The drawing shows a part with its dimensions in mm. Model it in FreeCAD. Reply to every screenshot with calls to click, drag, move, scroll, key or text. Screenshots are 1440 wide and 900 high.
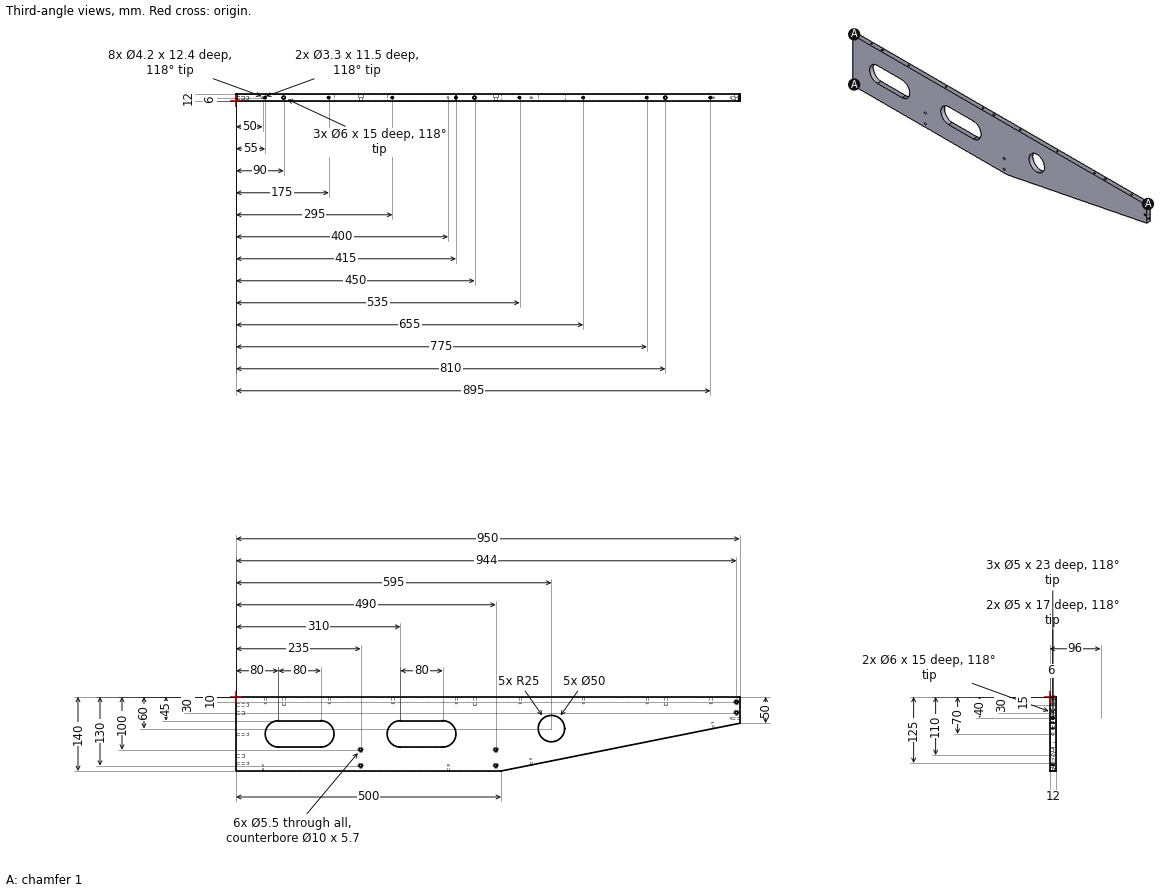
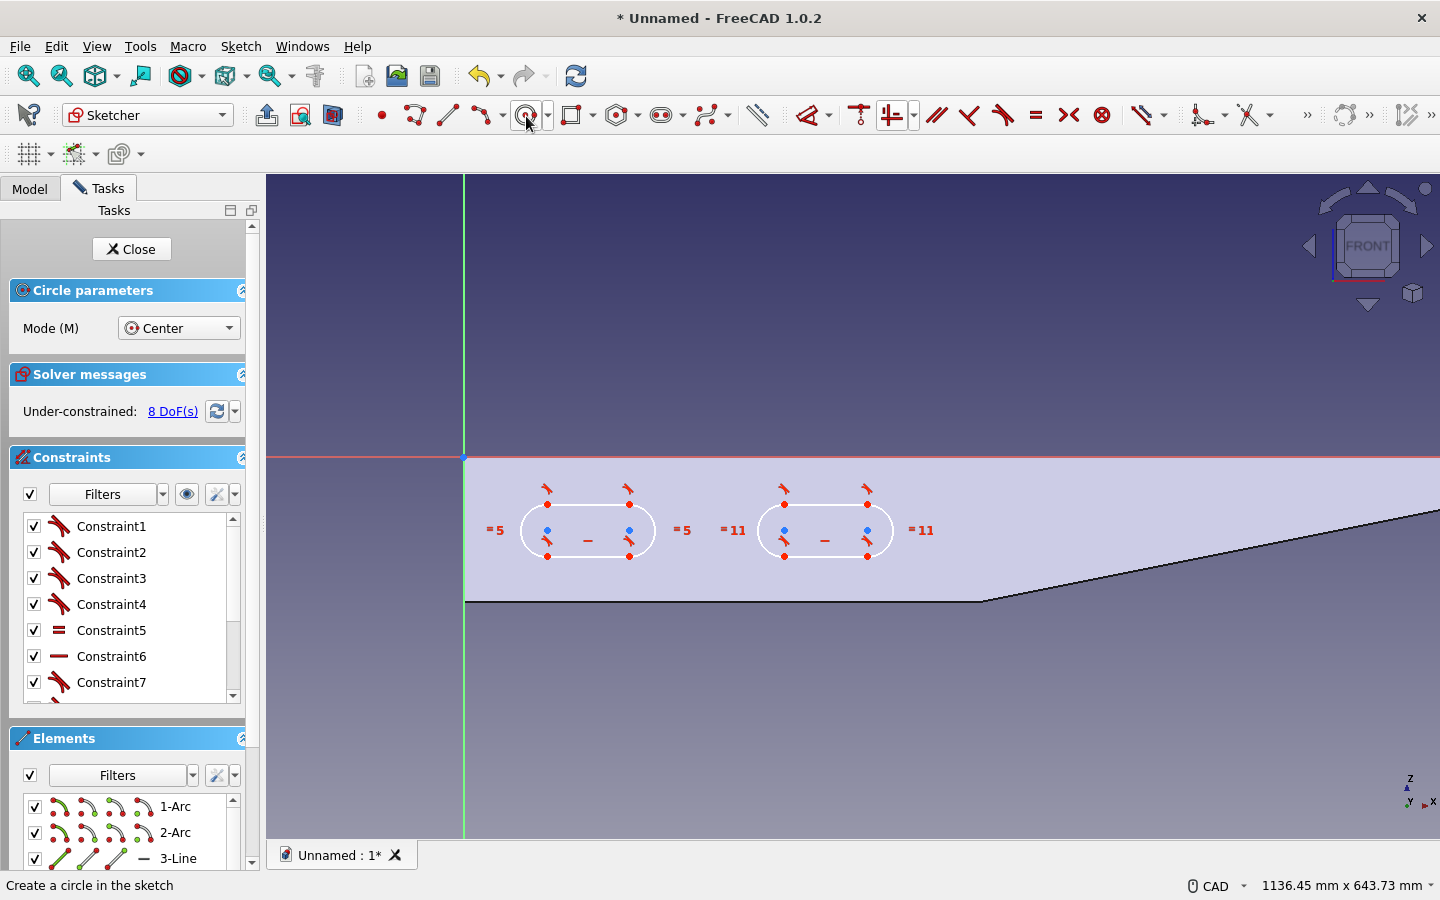
click(1079, 519)
move(1097, 501)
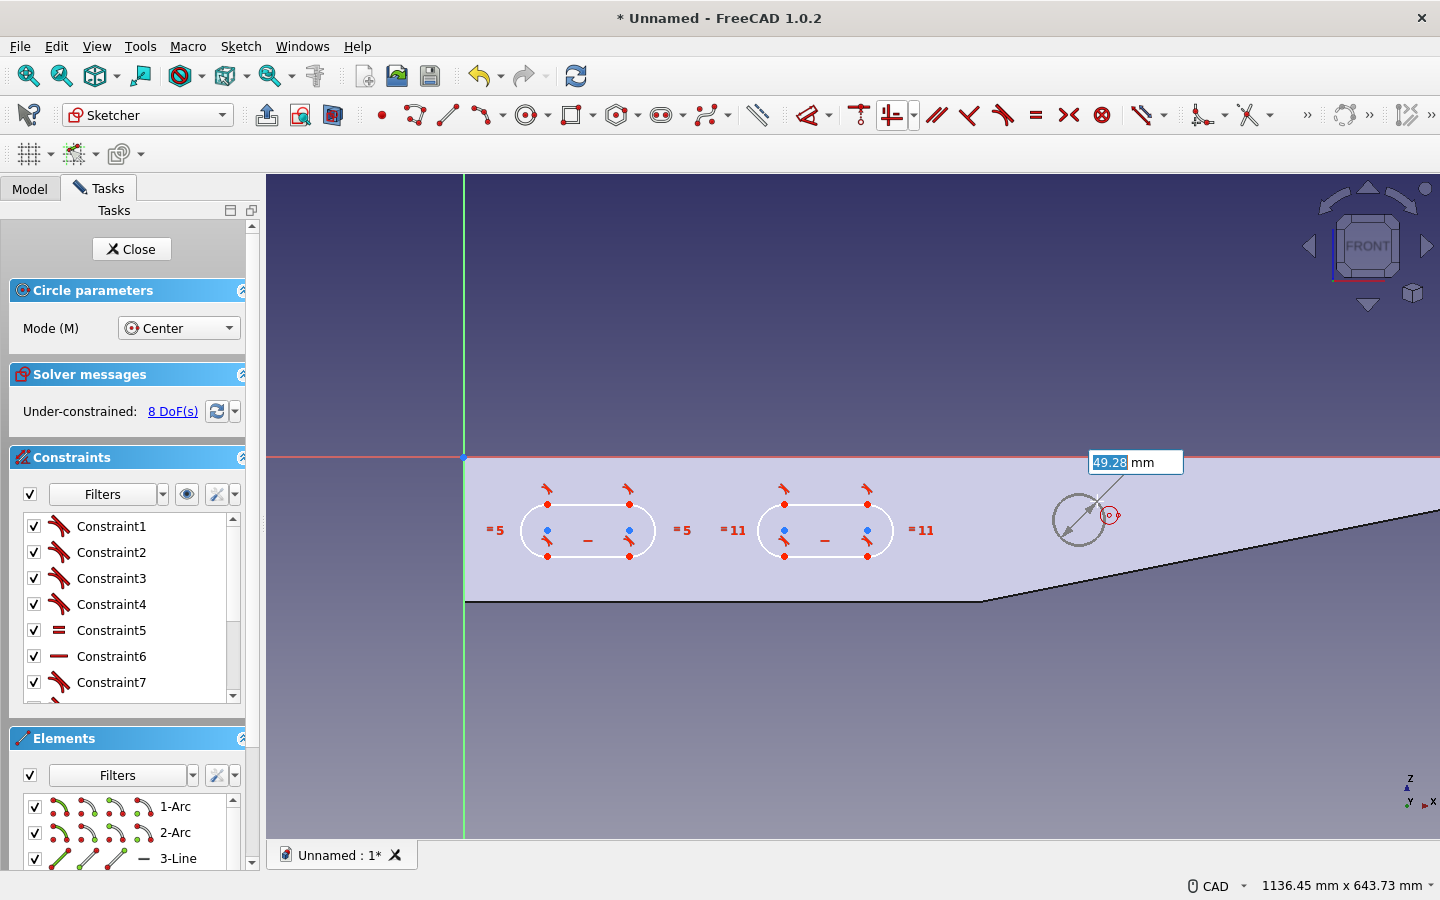
text(50)
key(Return)
key(Escape)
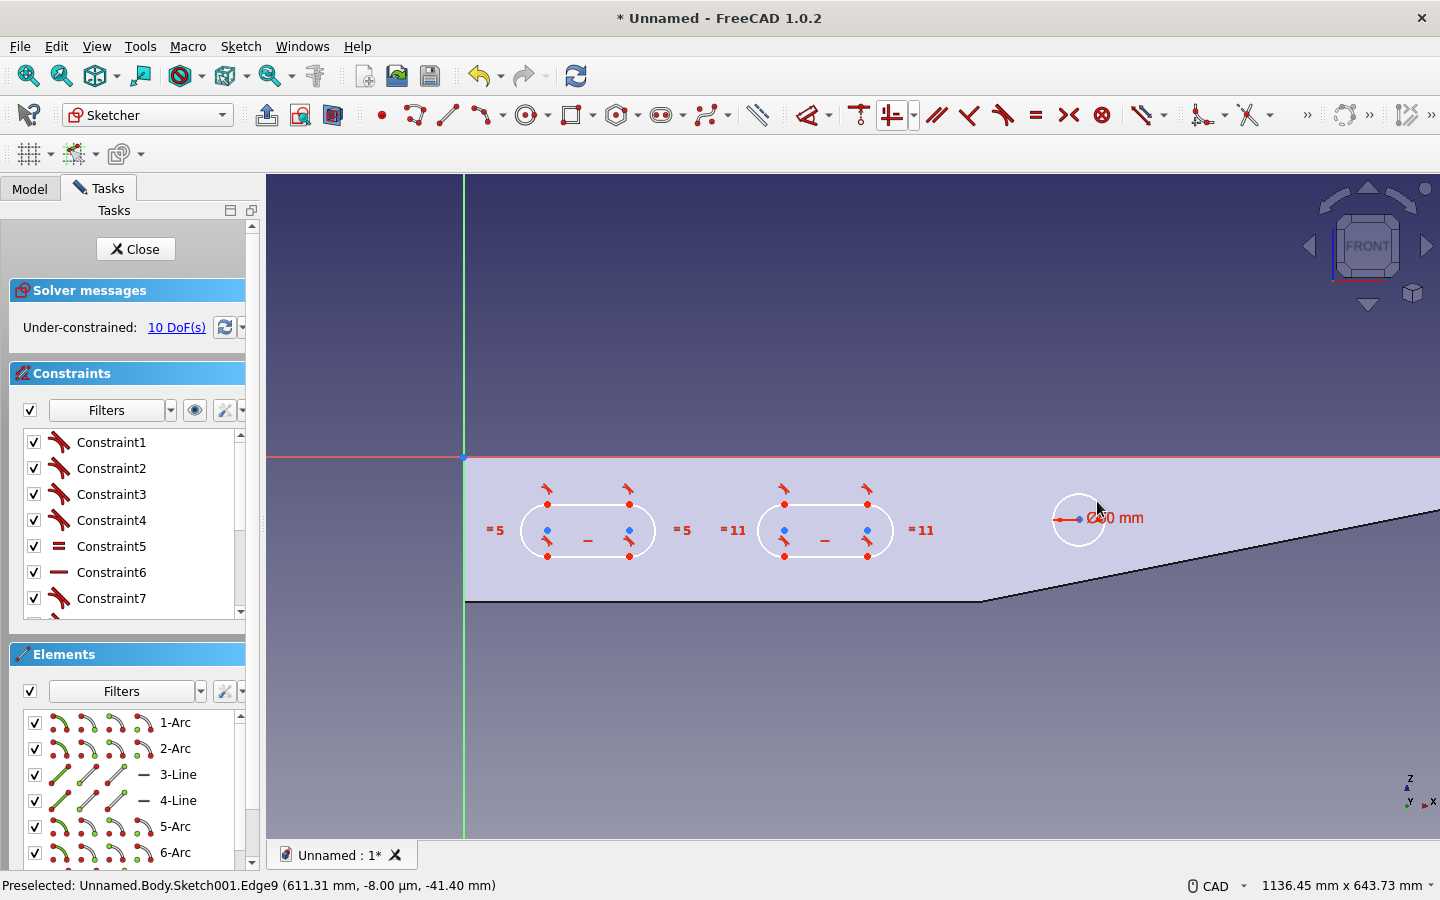
click(526, 516)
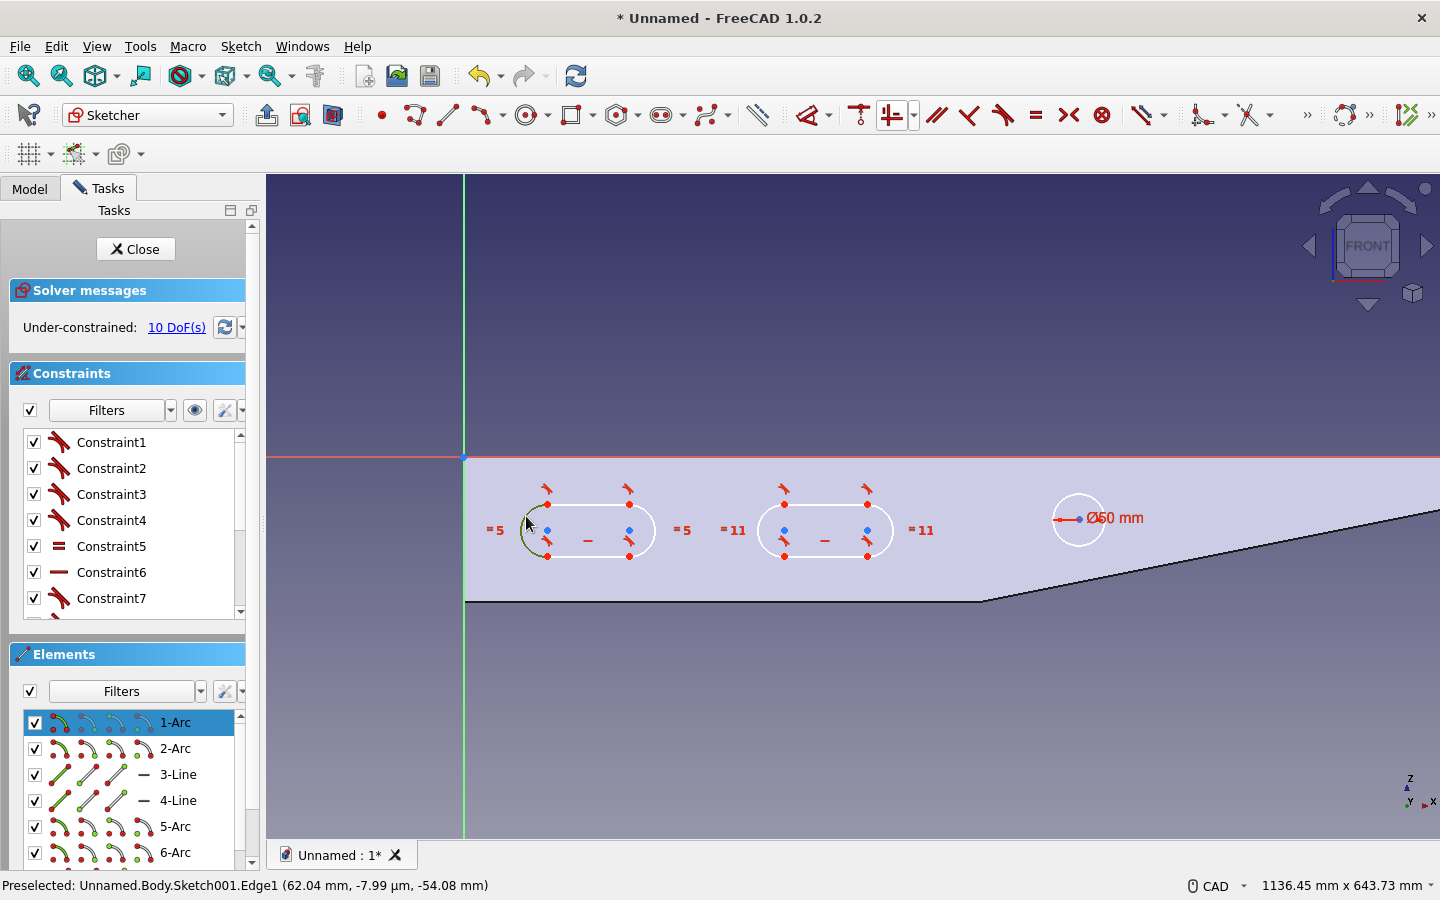
click(763, 516)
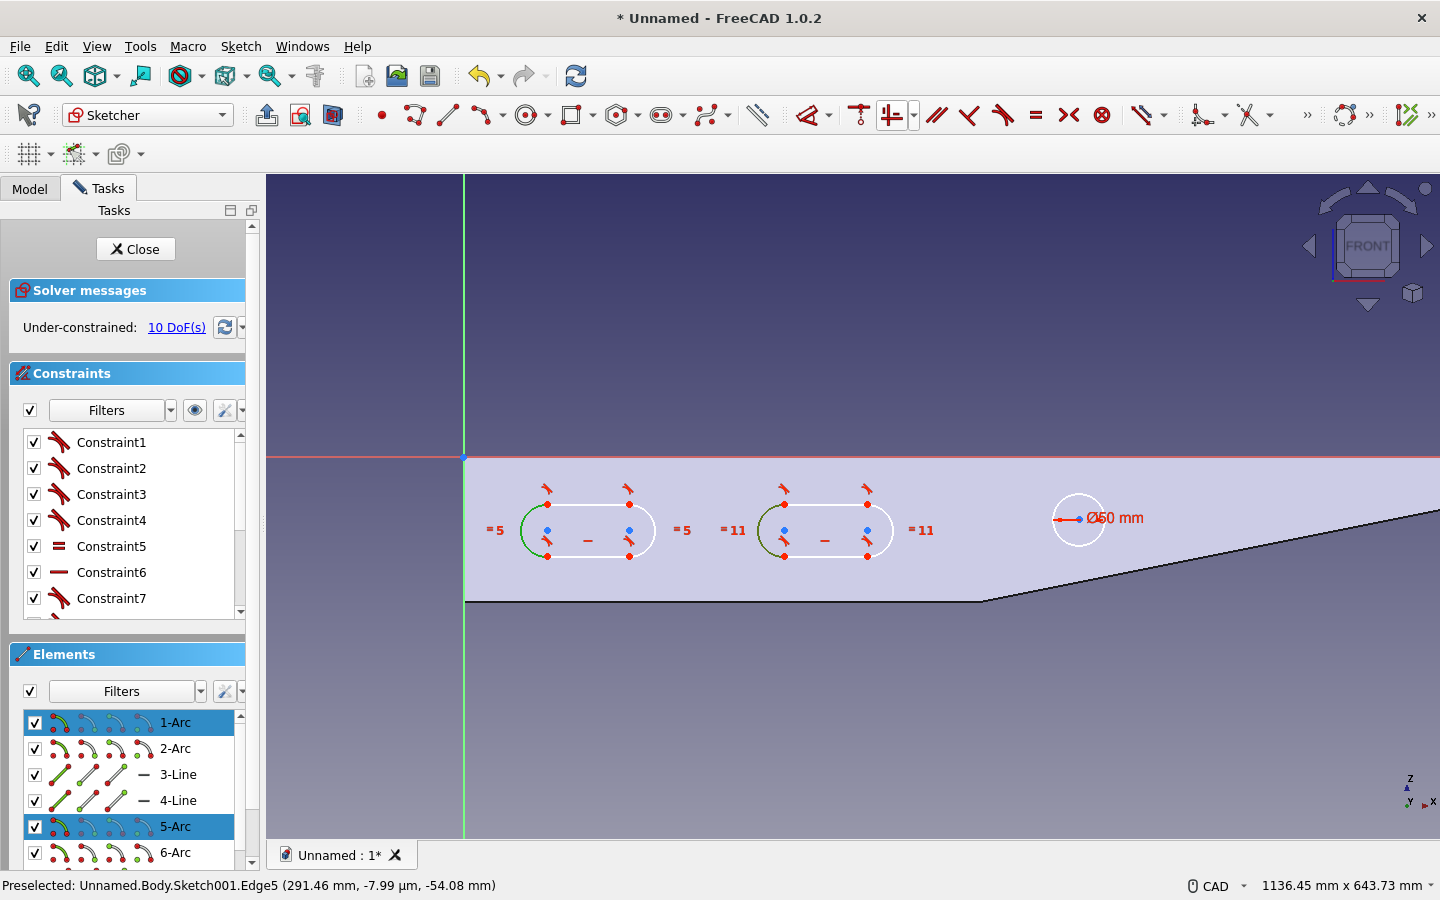
key(e)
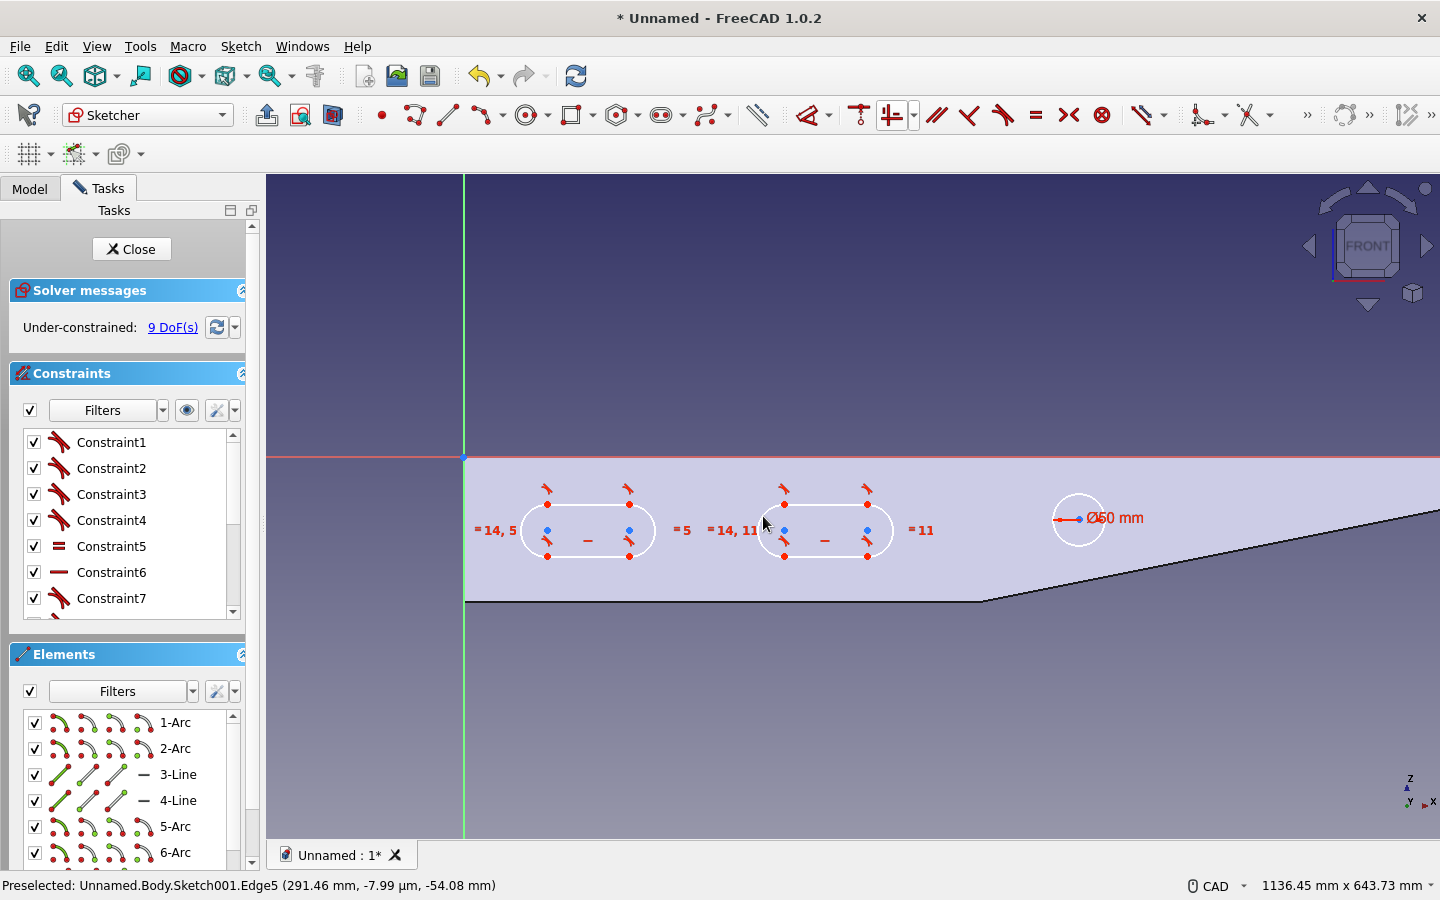
click(806, 116)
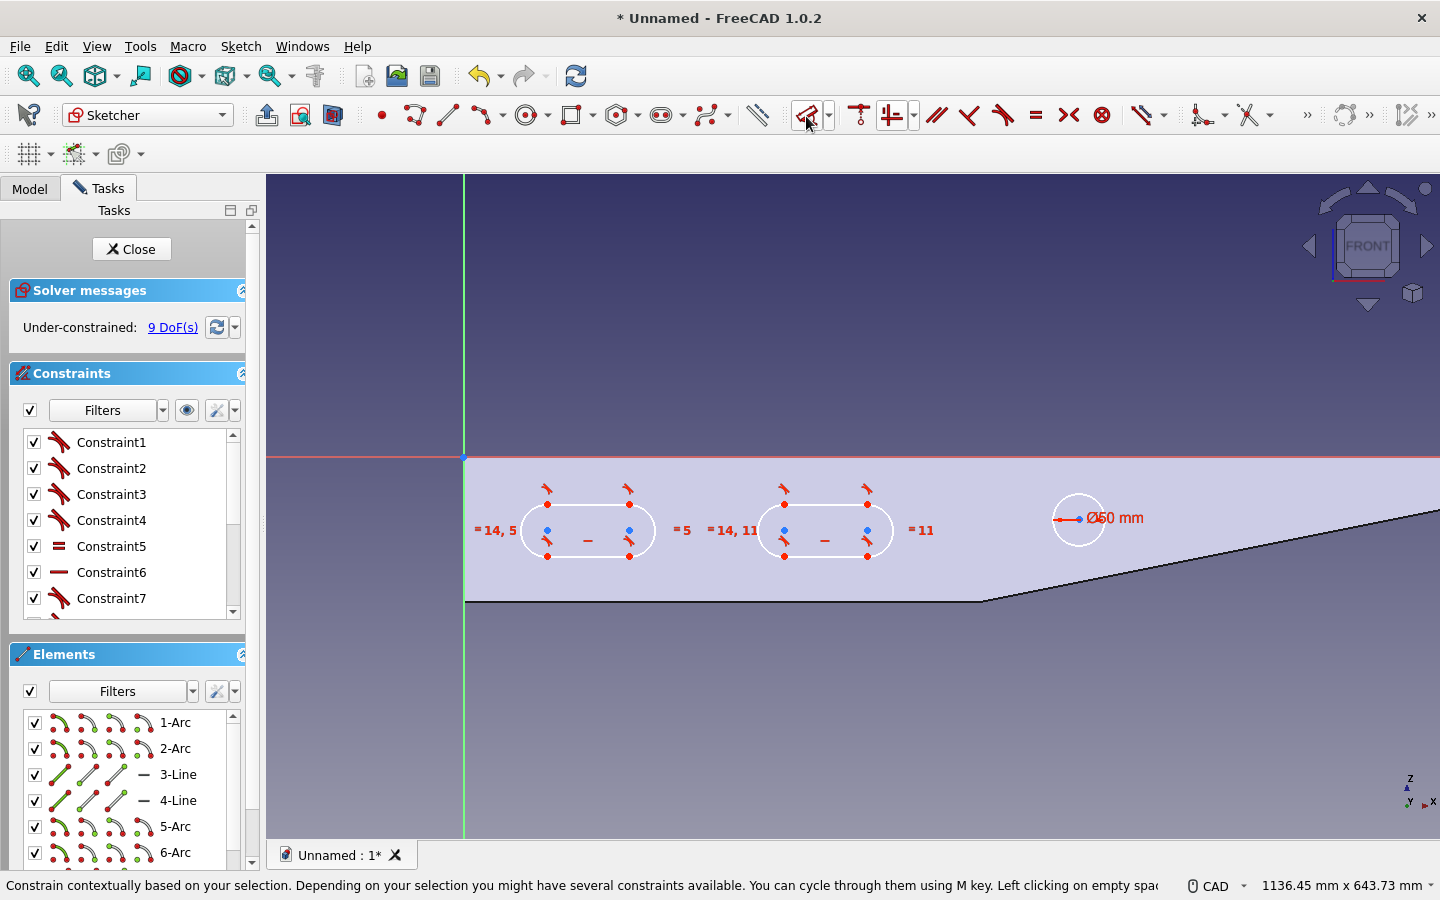
scroll(526, 516, up, 3)